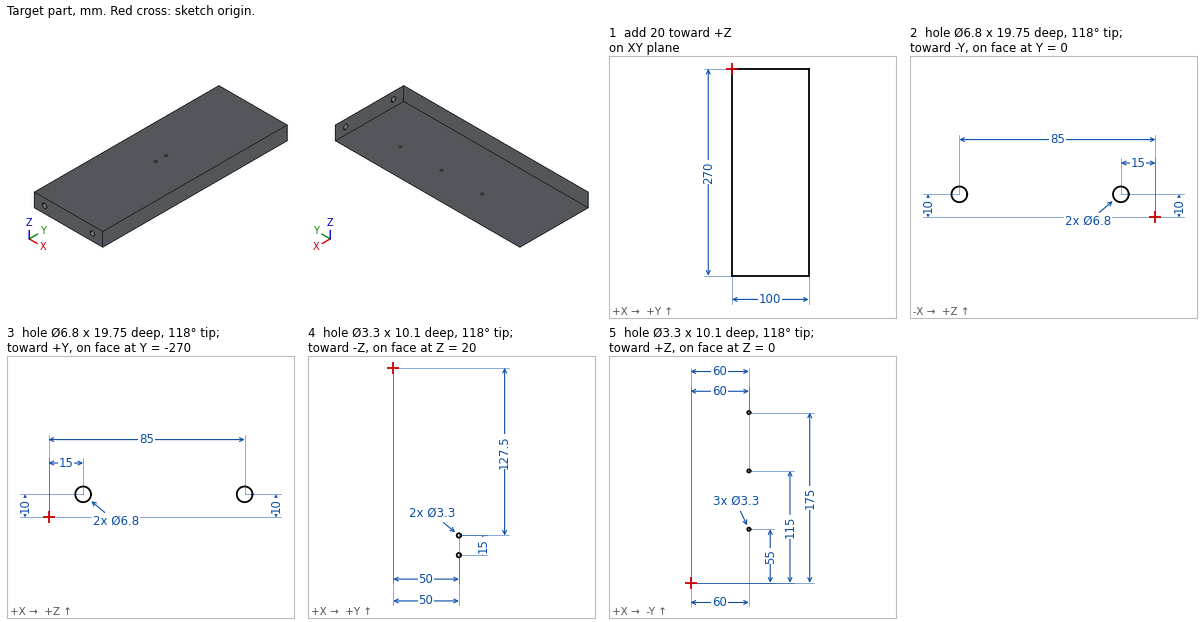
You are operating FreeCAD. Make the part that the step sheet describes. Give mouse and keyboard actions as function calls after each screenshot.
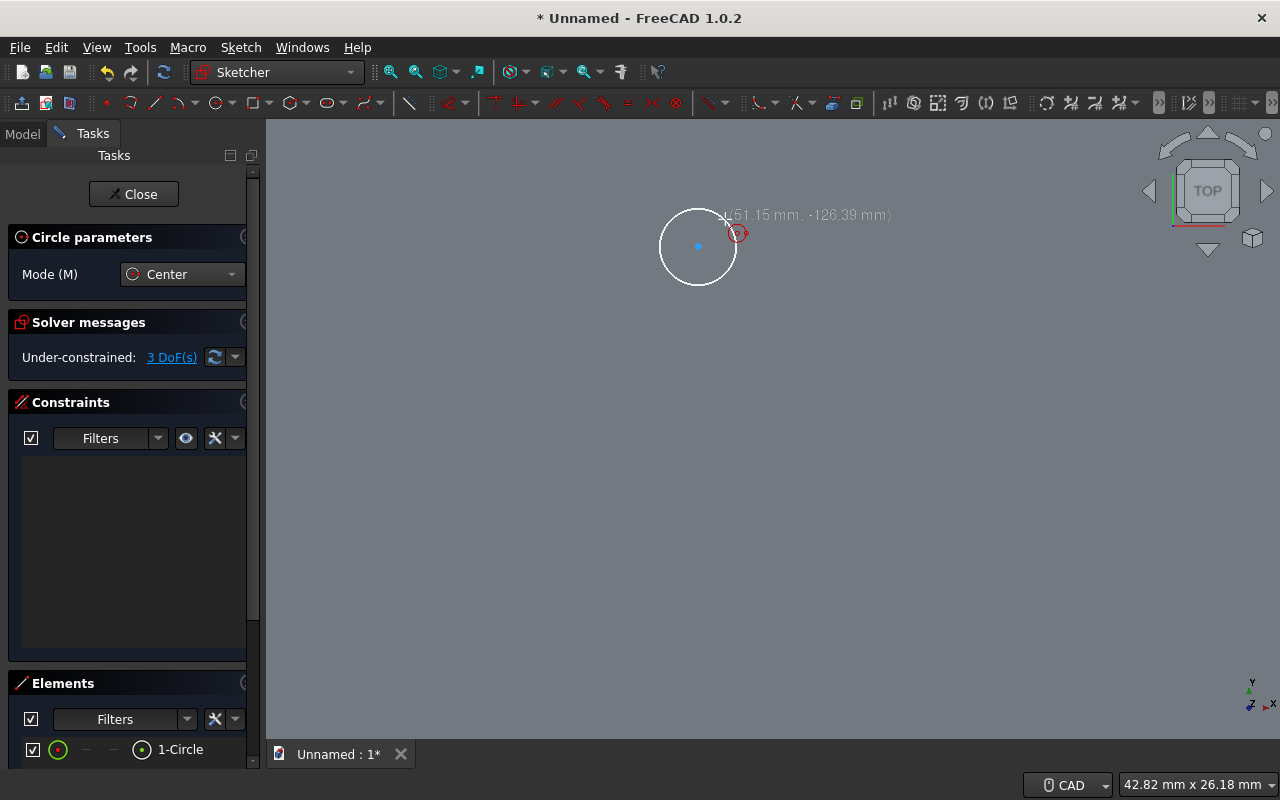
click(698, 602)
click(725, 574)
key(Escape)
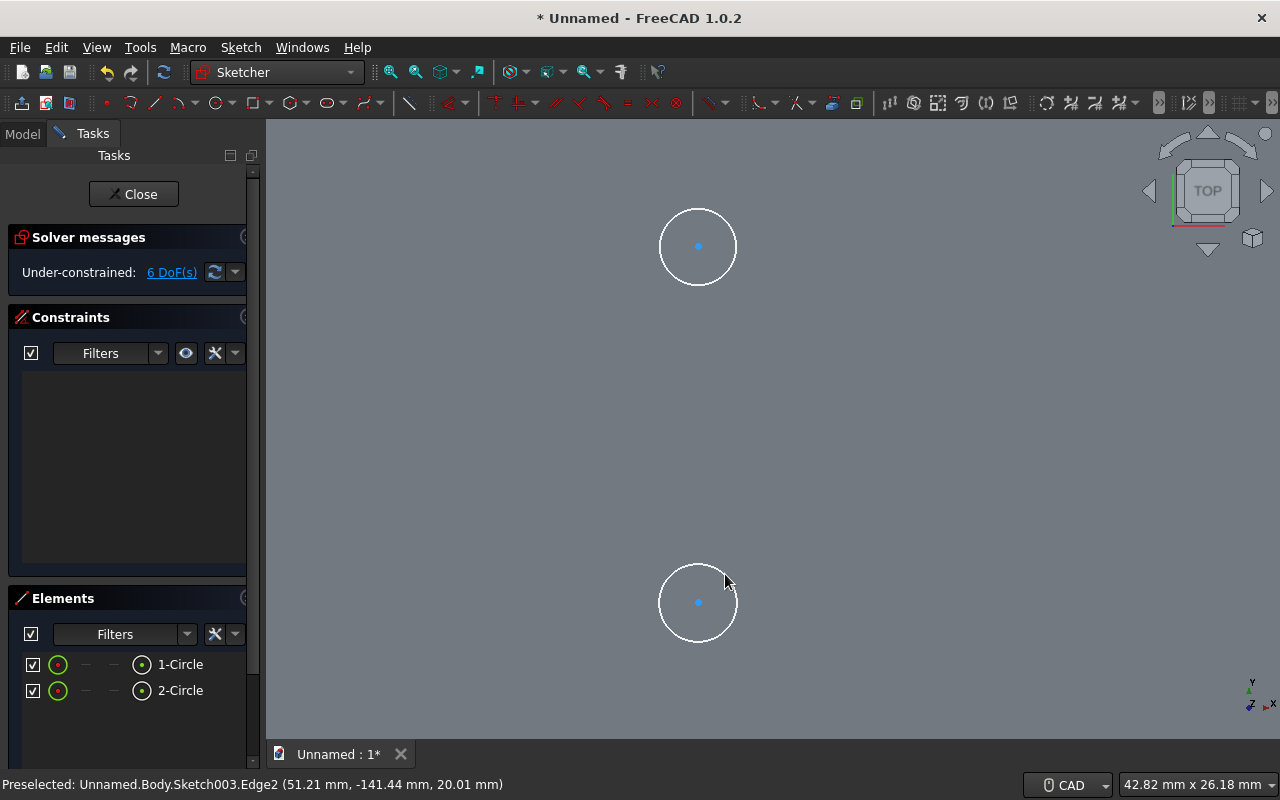
click(725, 220)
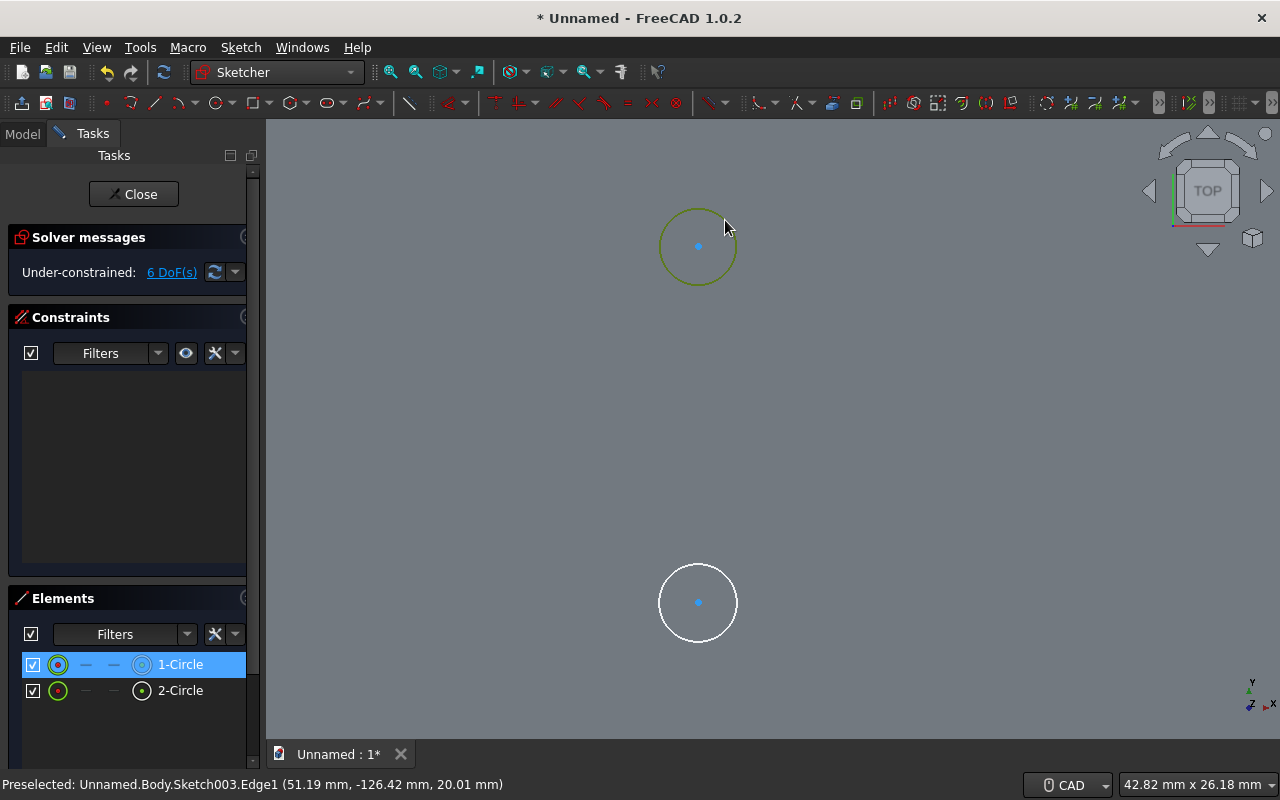
click(725, 575)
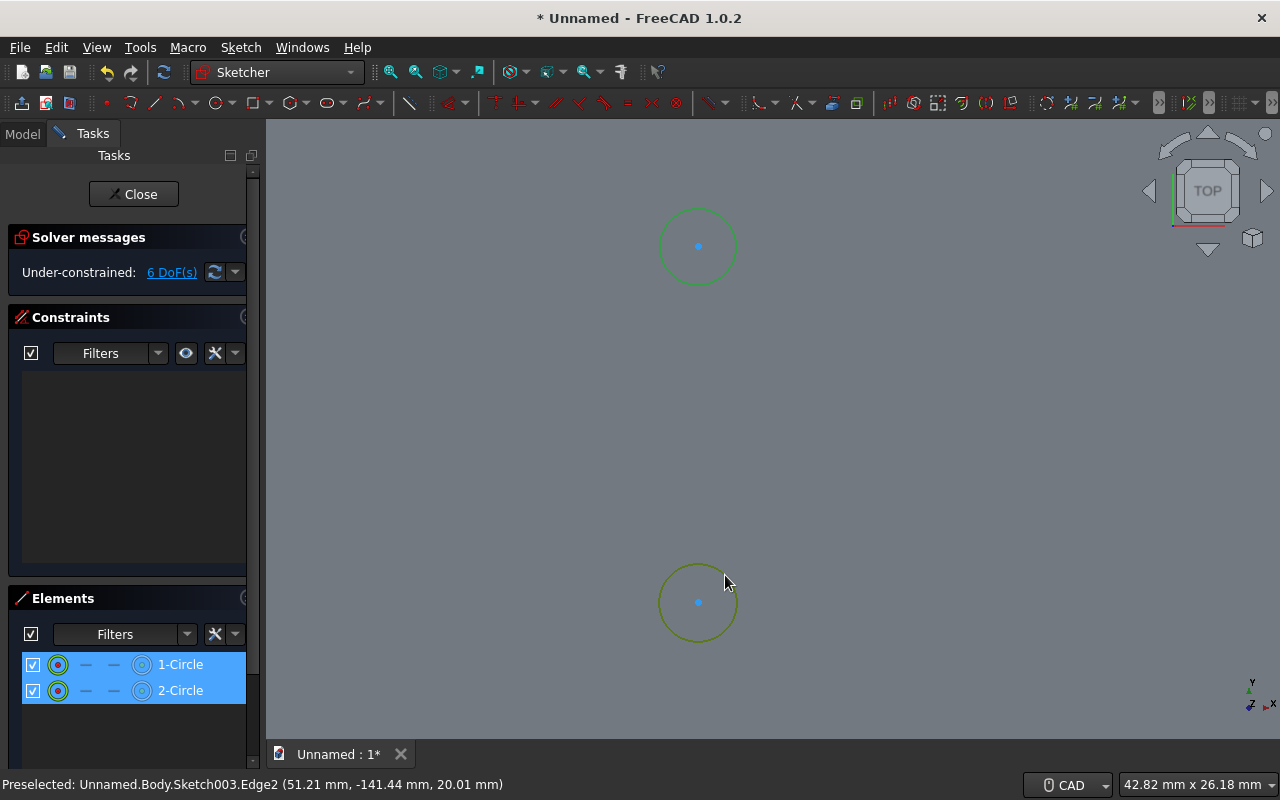
key(e)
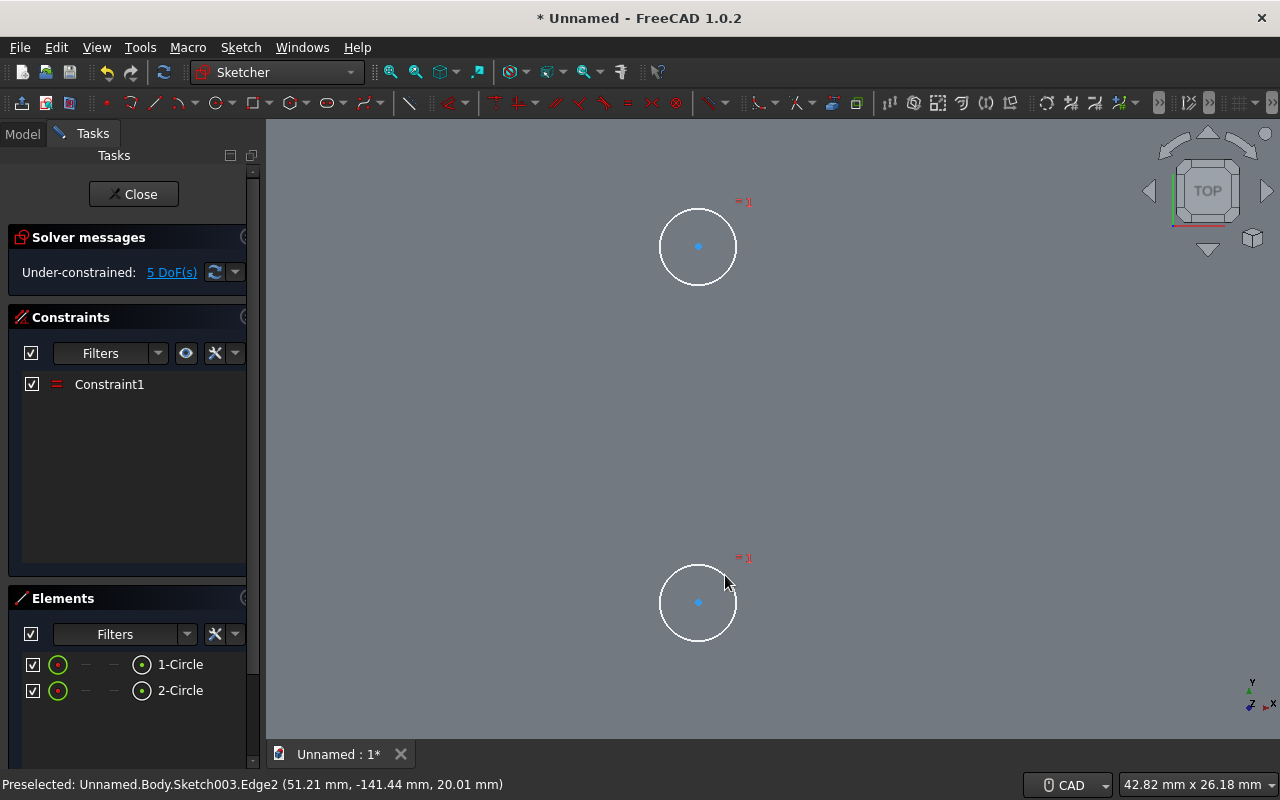
key(d)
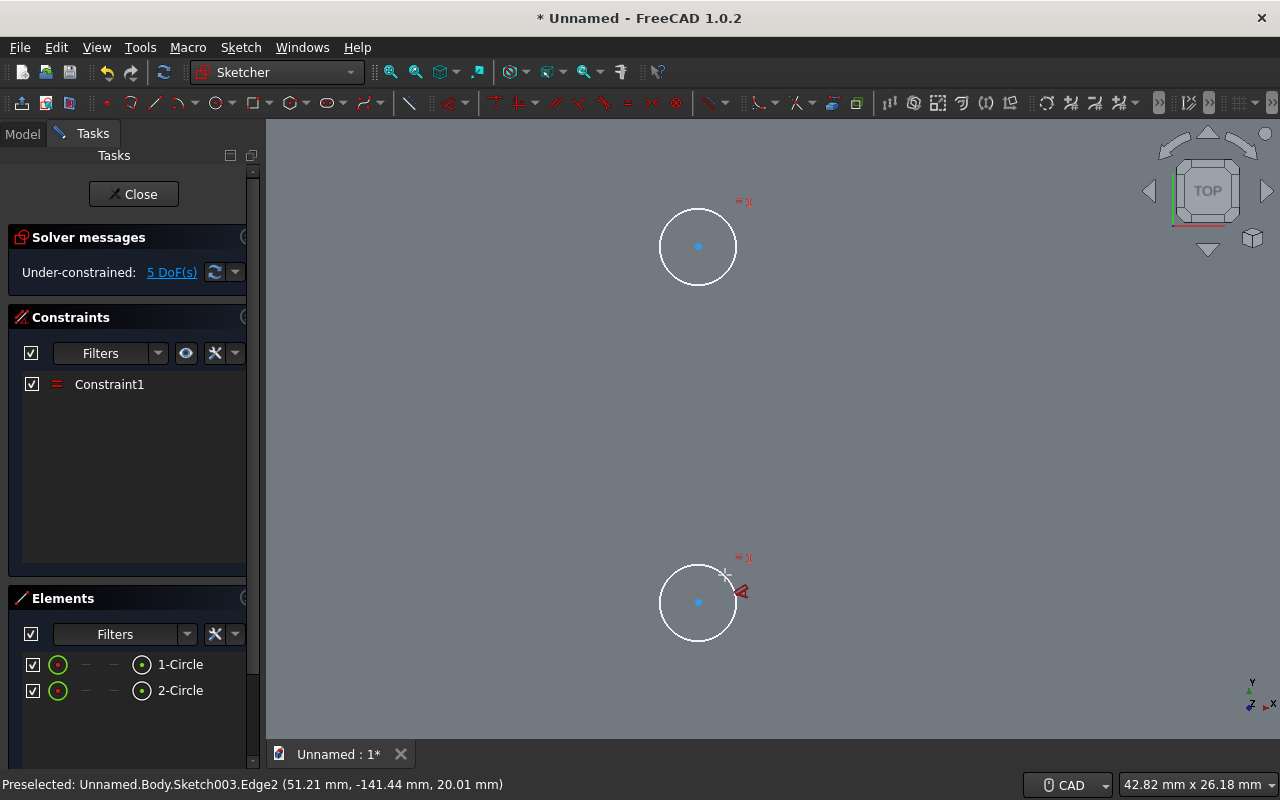
click(725, 220)
click(748, 197)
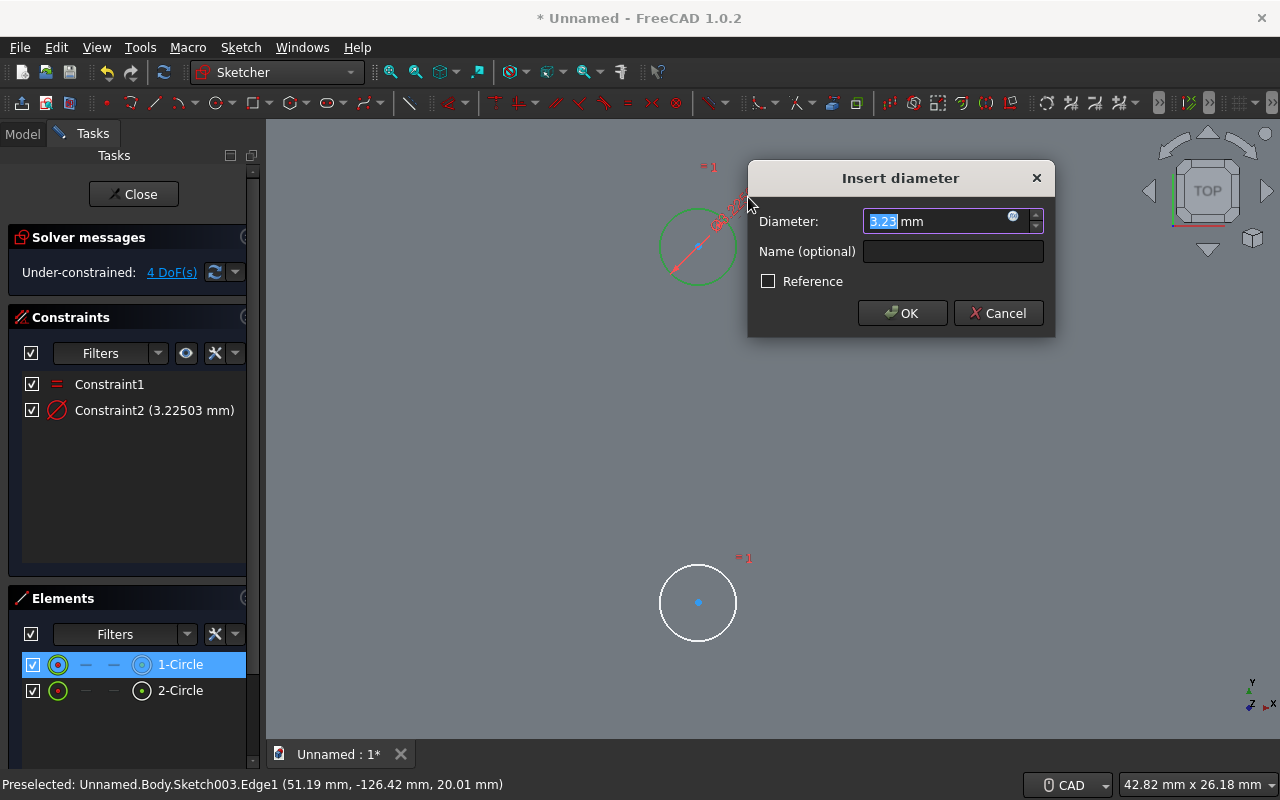
text(3.3)
key(Return)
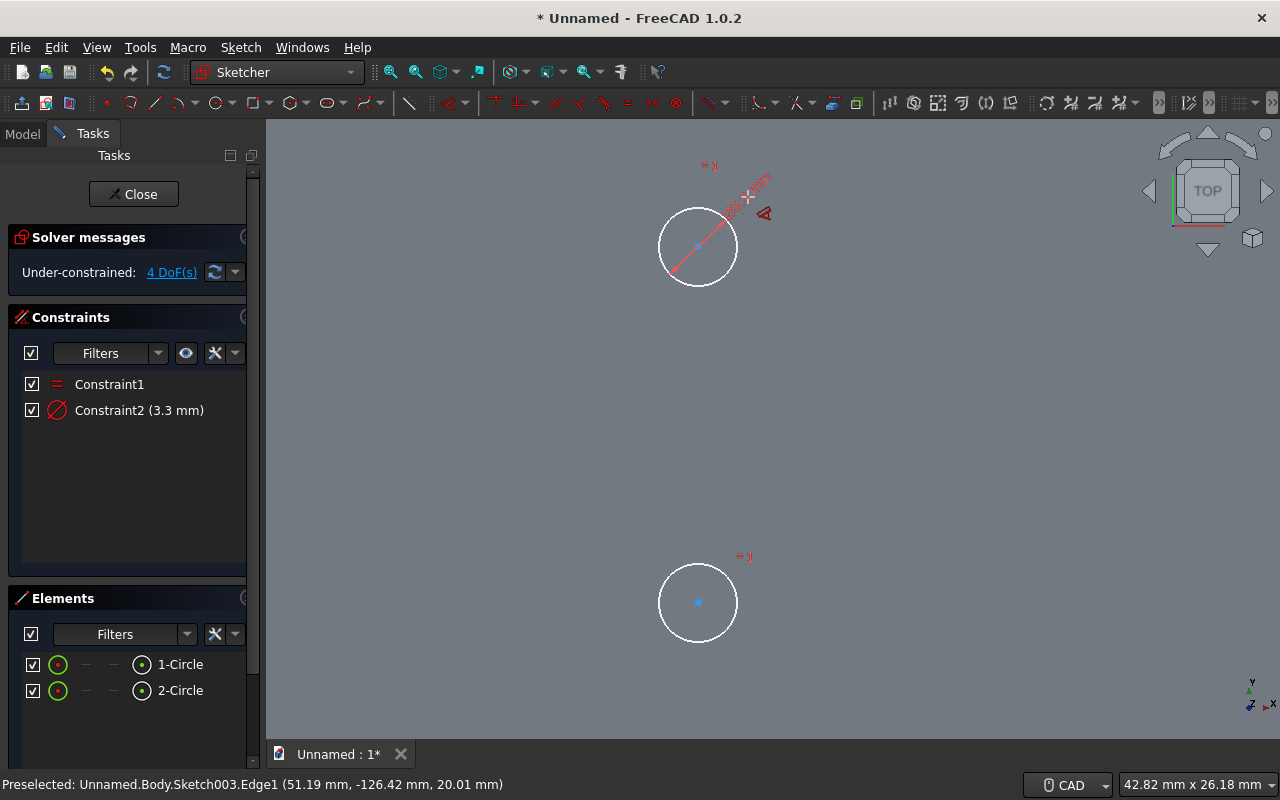
click(698, 247)
click(496, 281)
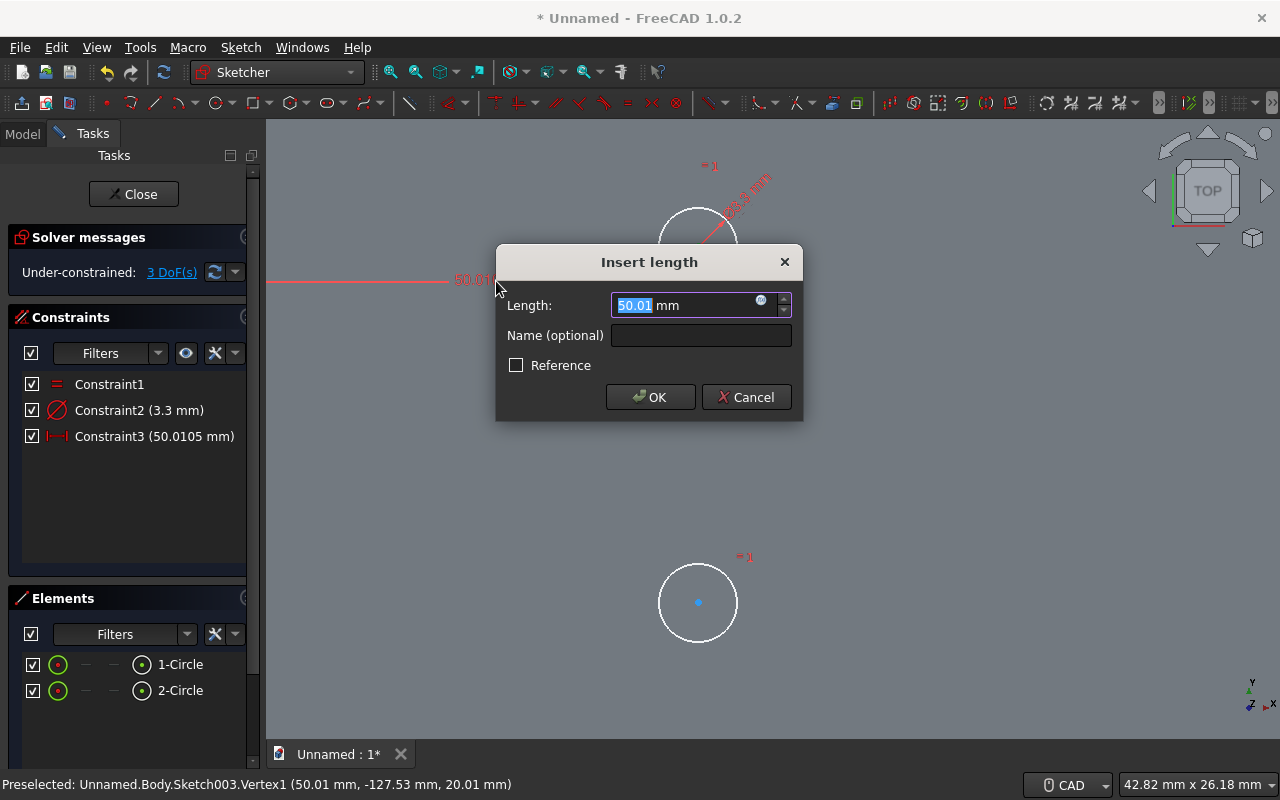
text(50)
key(Return)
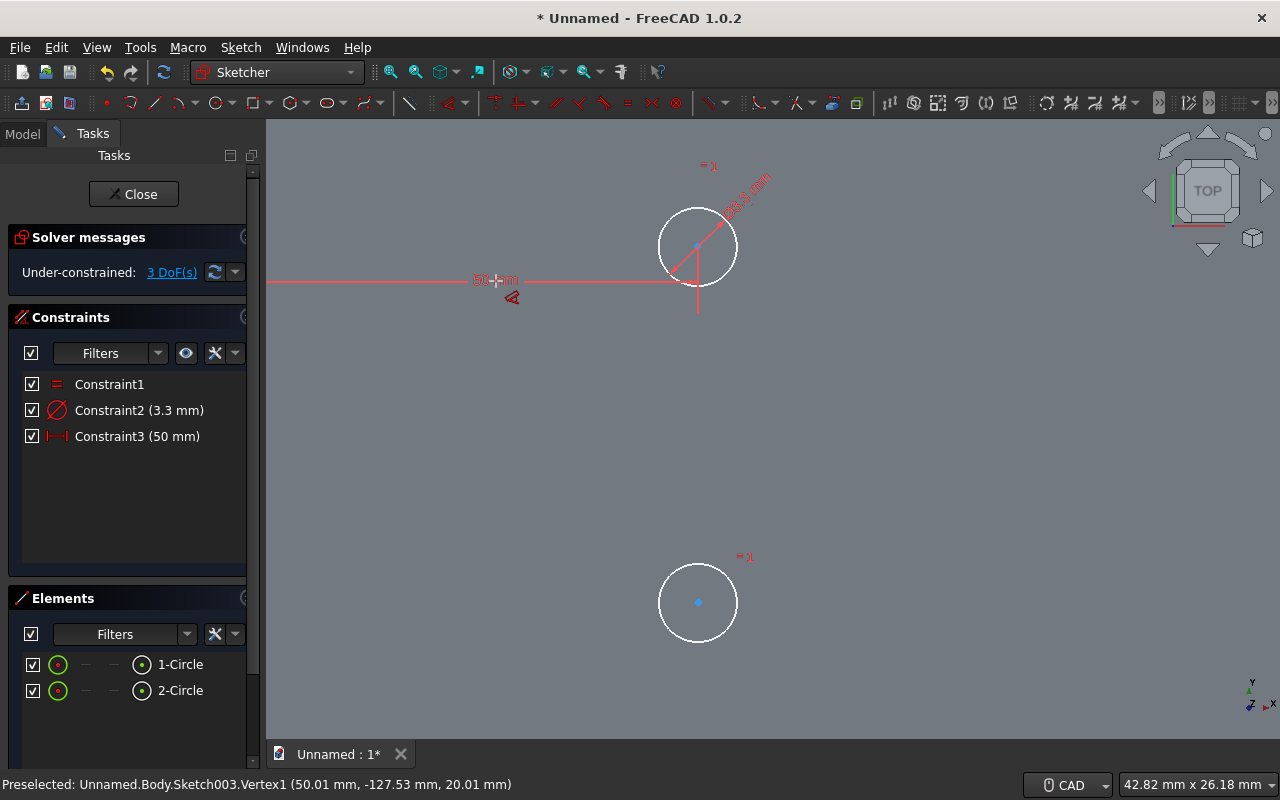
click(698, 603)
click(496, 637)